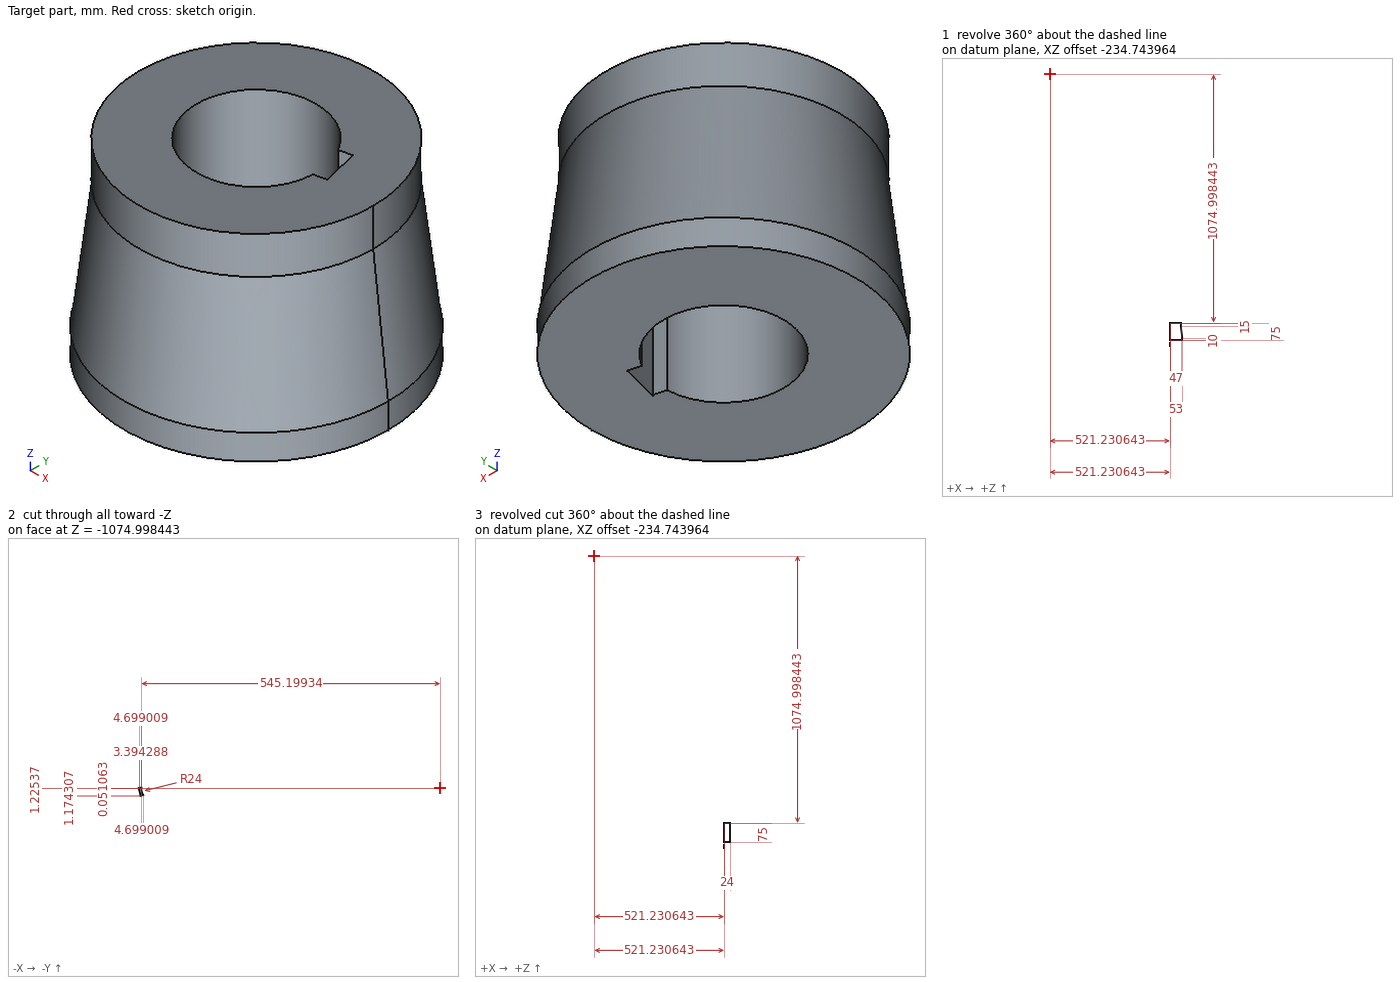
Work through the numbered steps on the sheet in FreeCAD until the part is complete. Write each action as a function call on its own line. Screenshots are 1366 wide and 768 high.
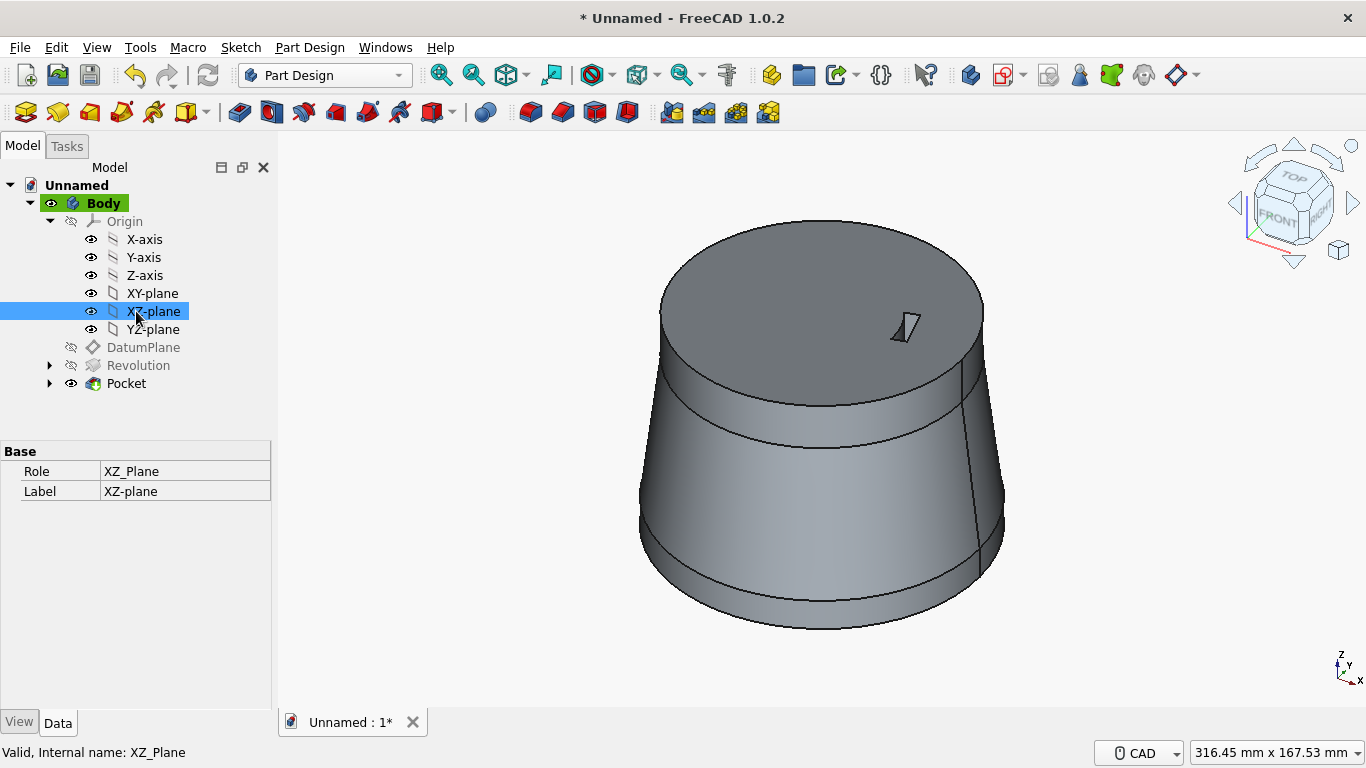
click(1176, 76)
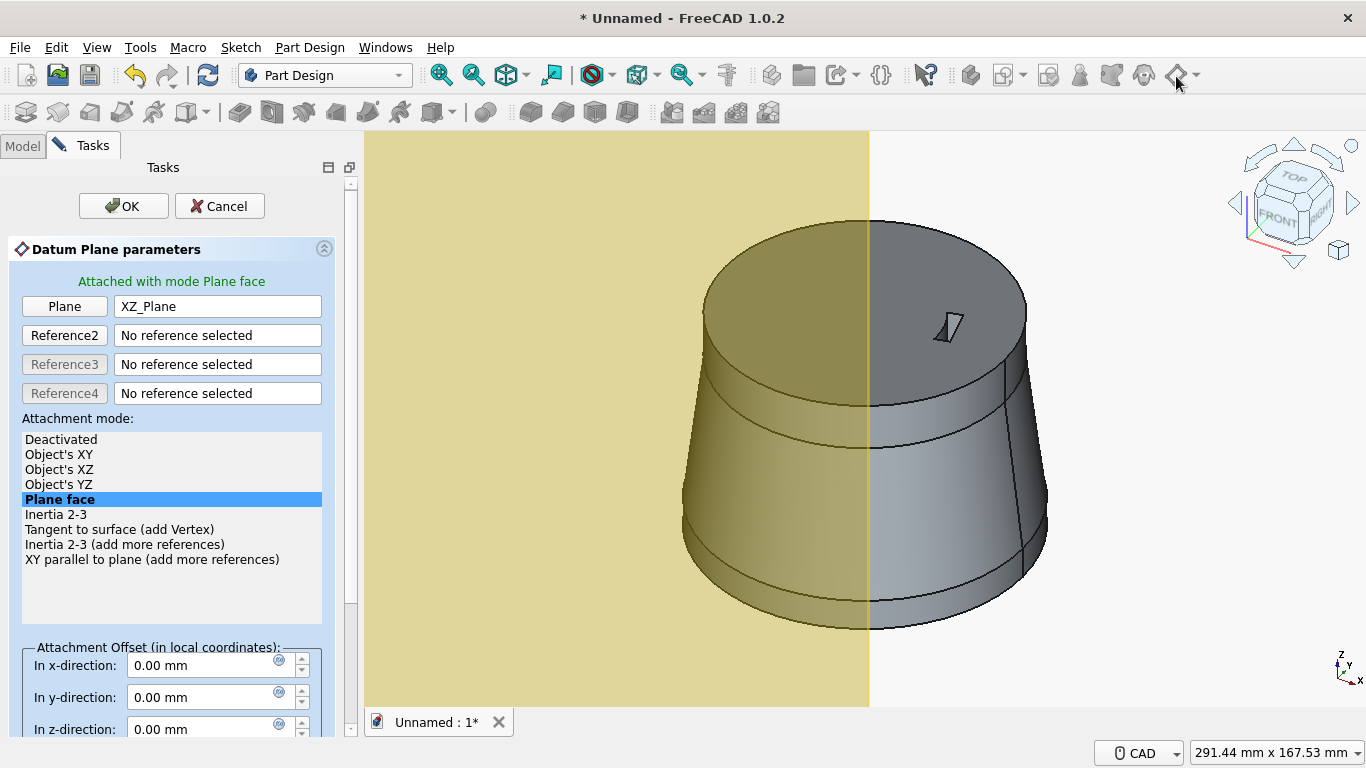
scroll(351, 456, down, 2)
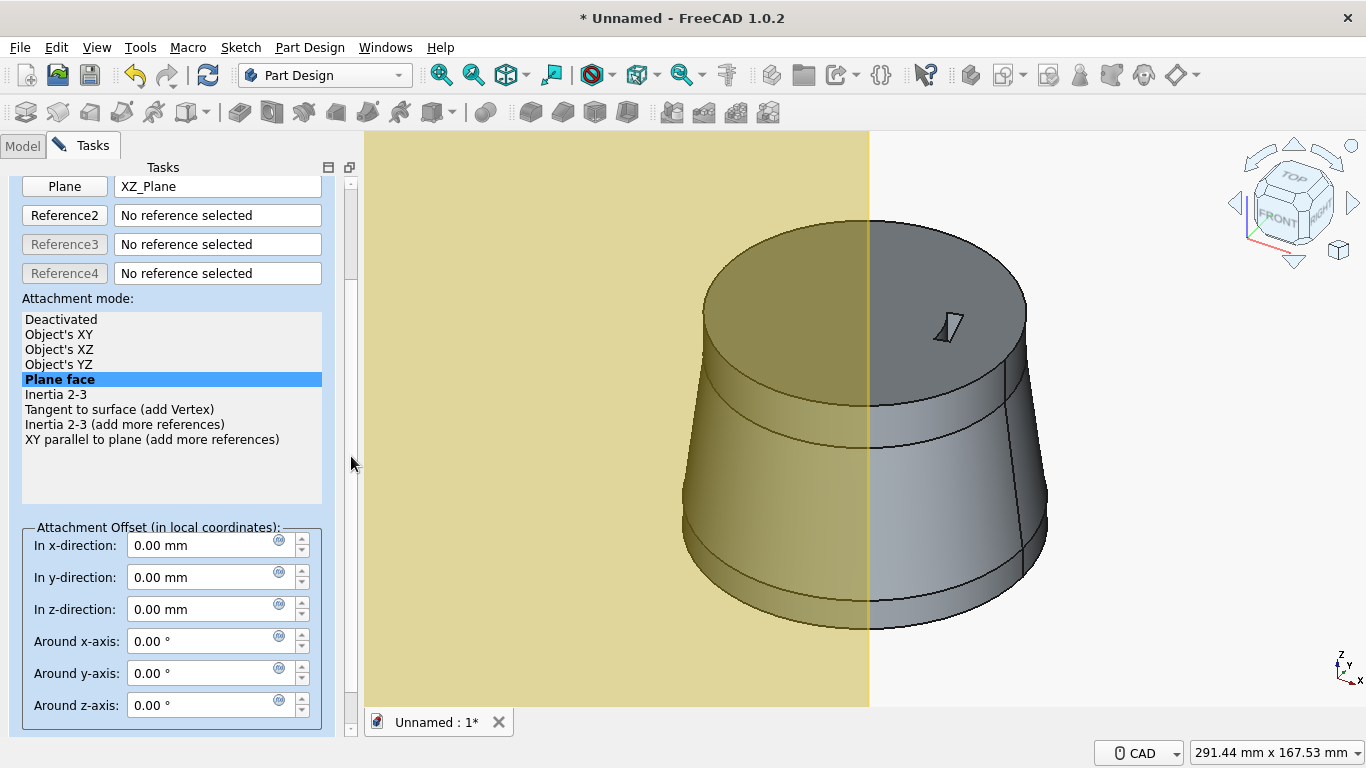
triple_click(210, 609)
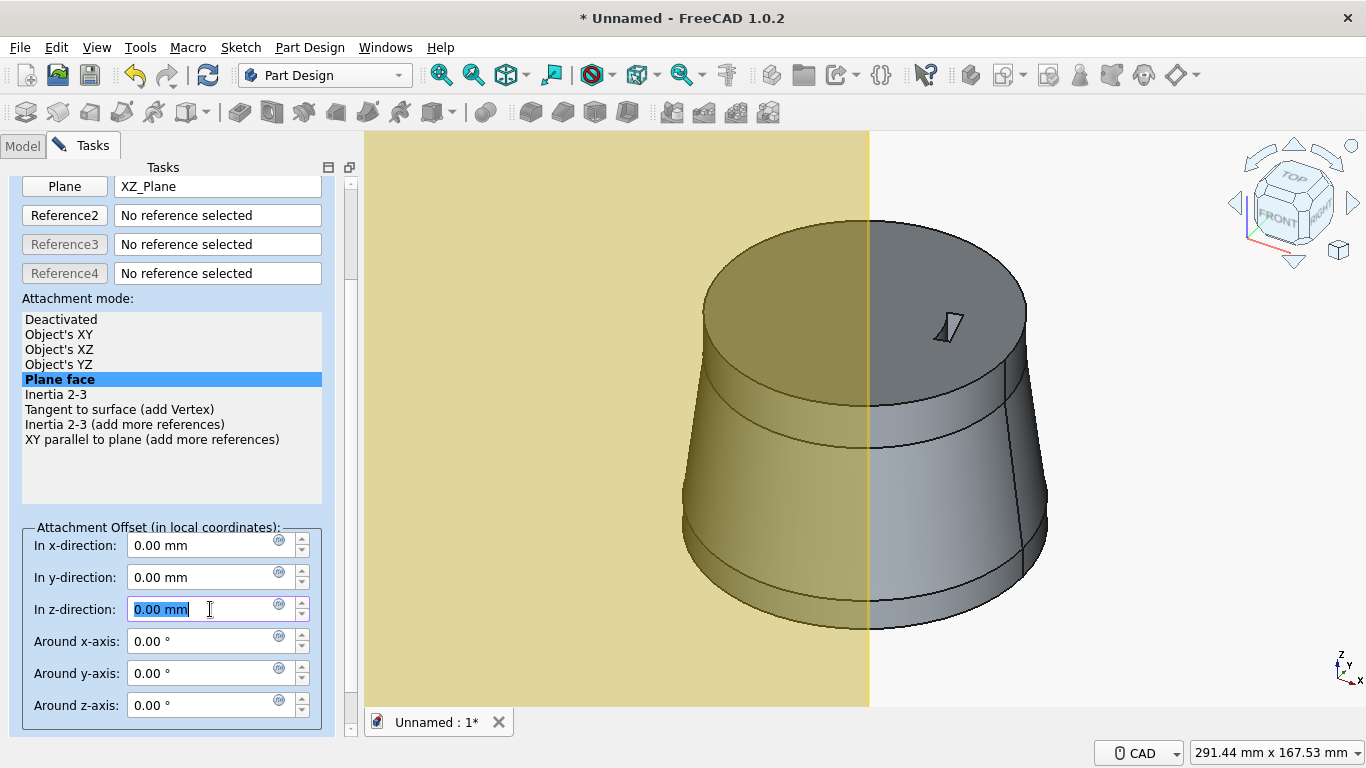
text(-234.743964)
key(Tab)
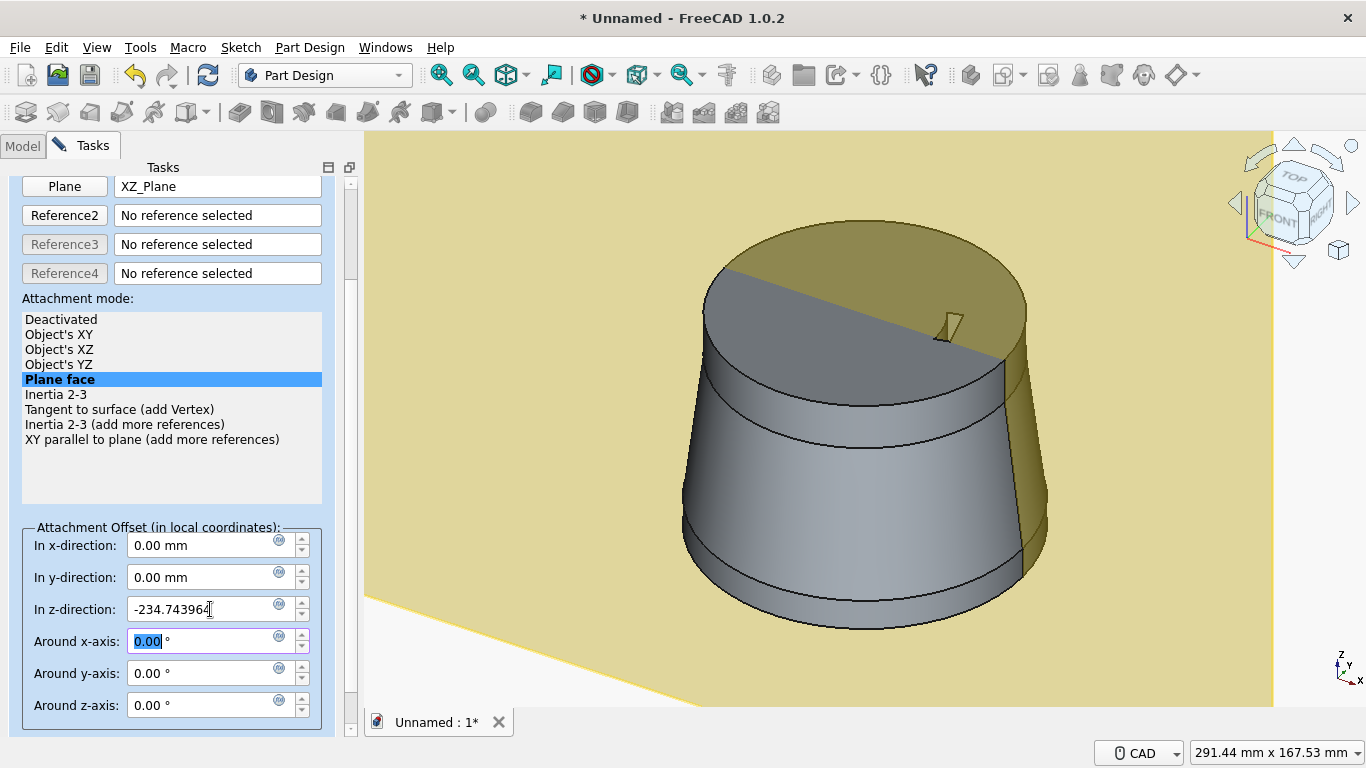
scroll(351, 456, up, 3)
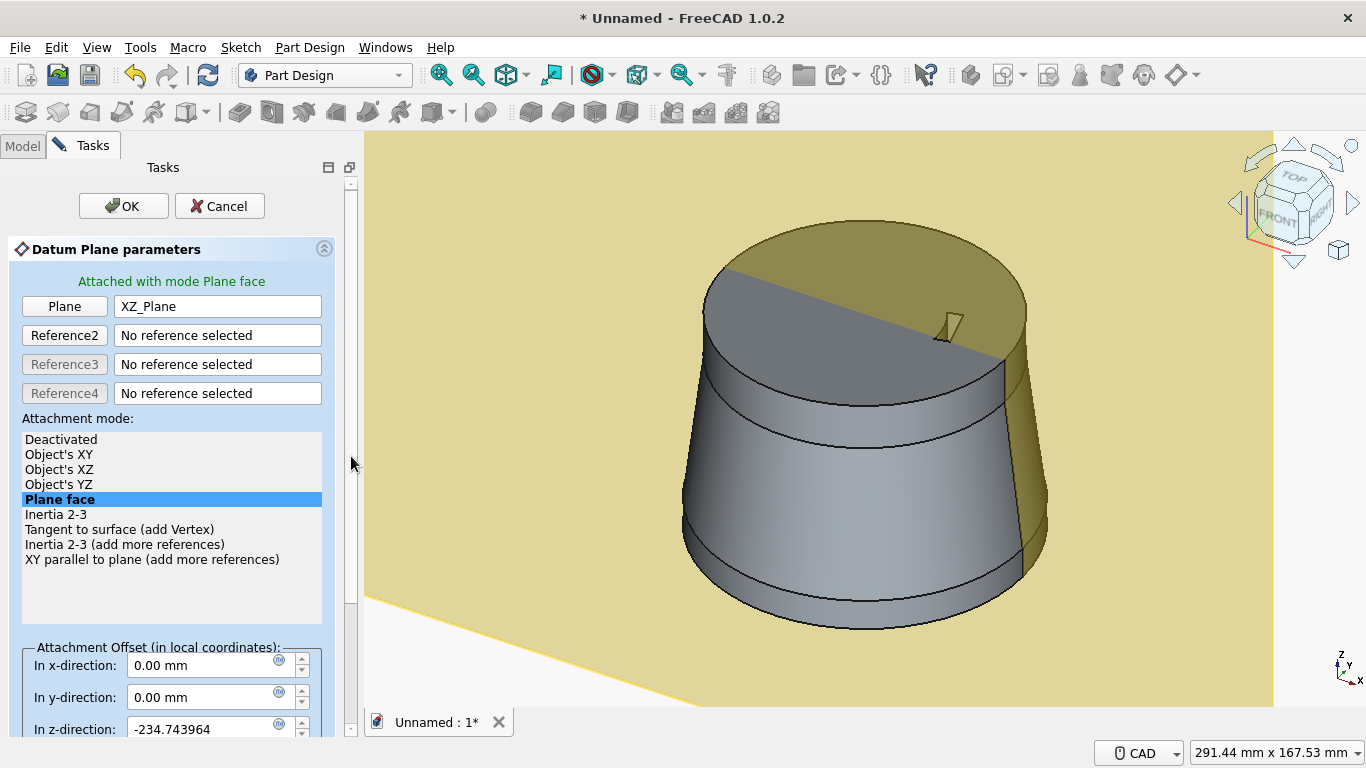
click(124, 206)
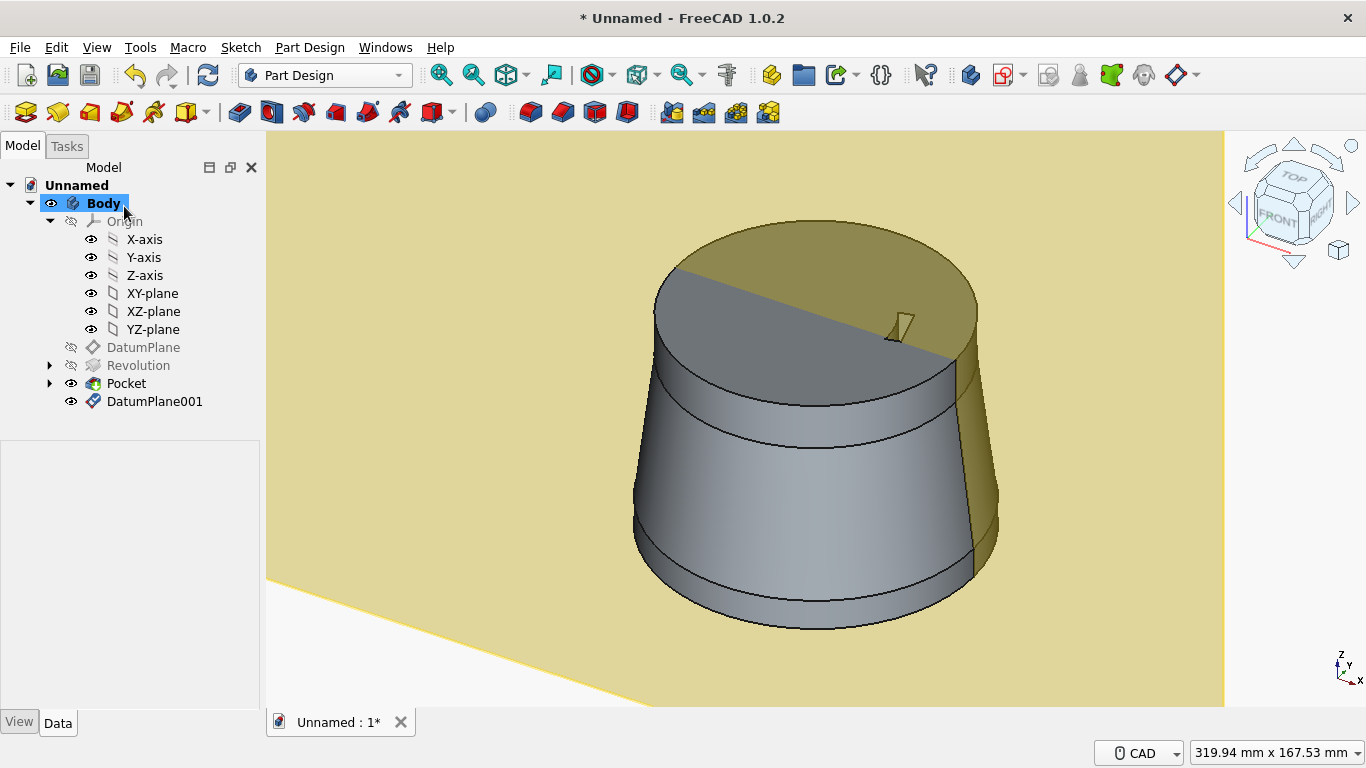
click(116, 401)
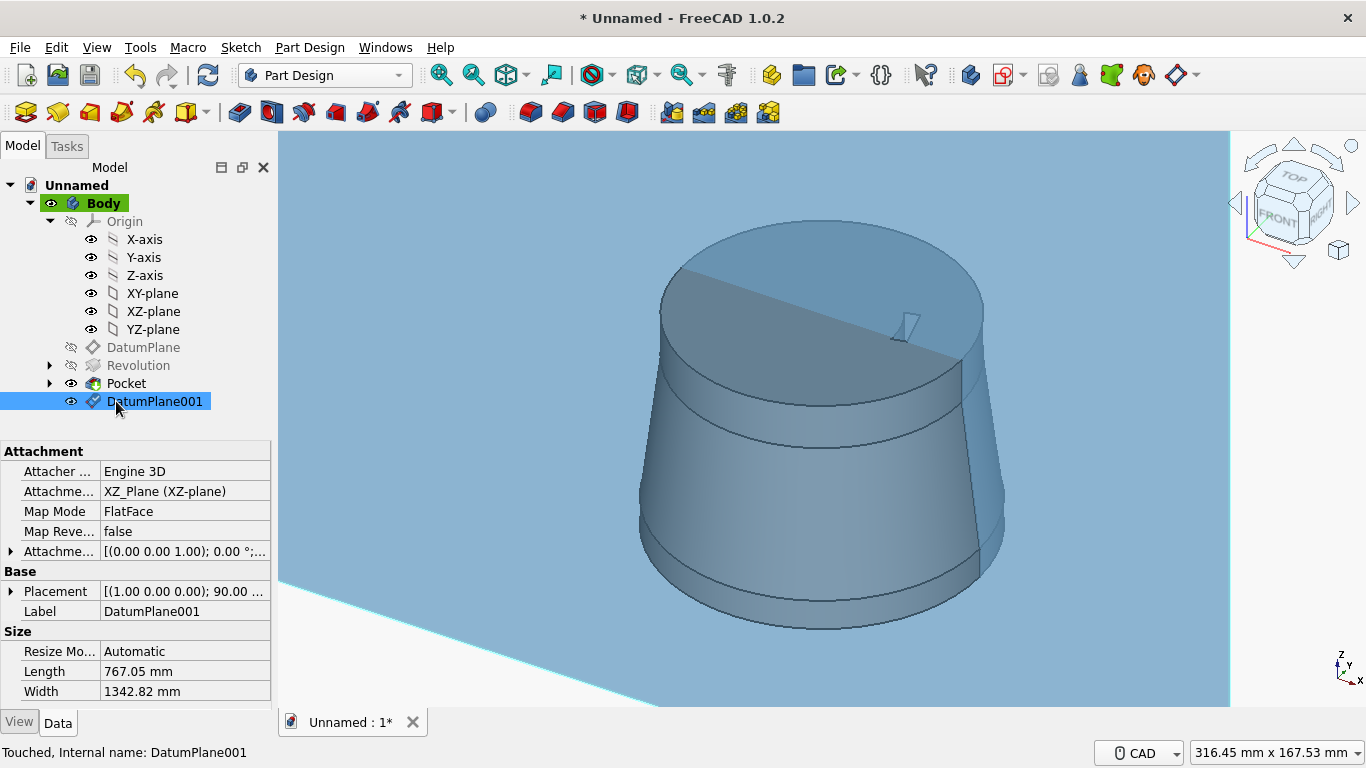
click(1004, 76)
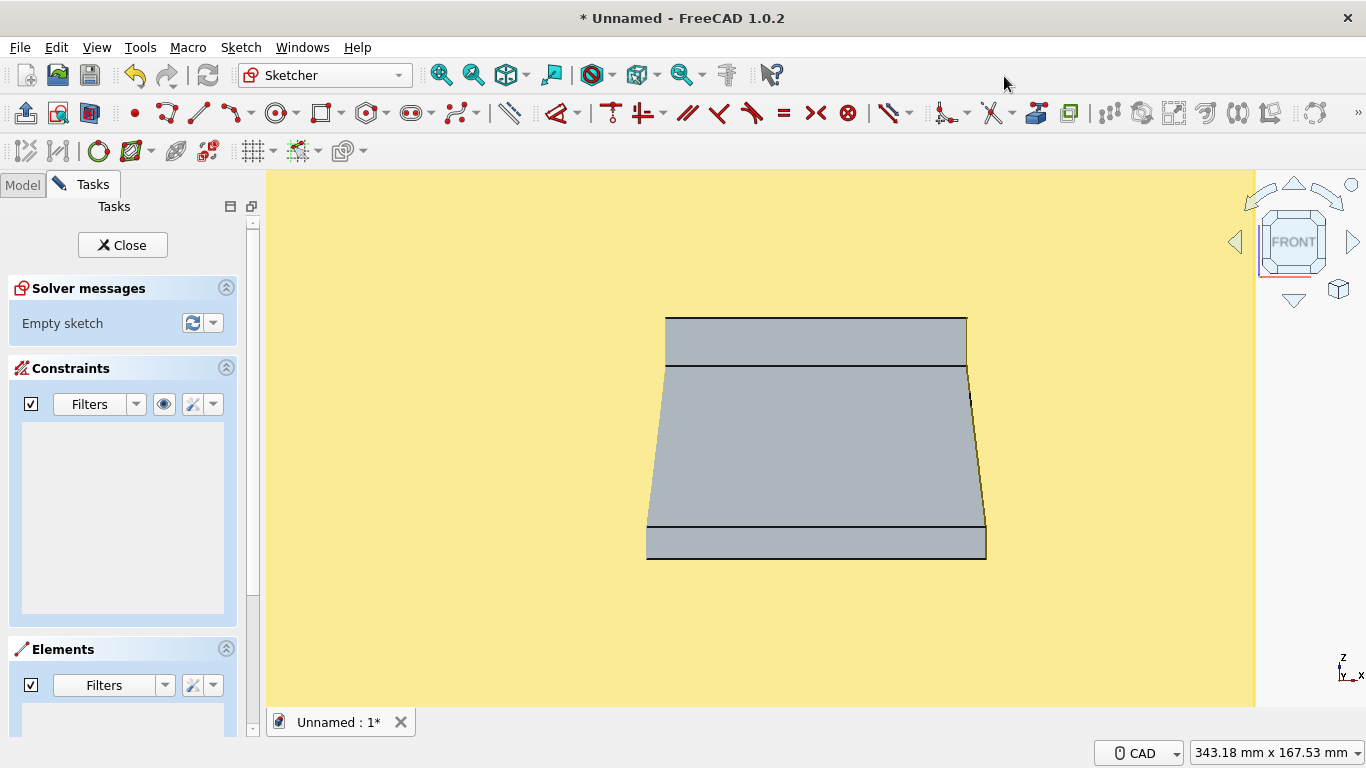
click(90, 114)